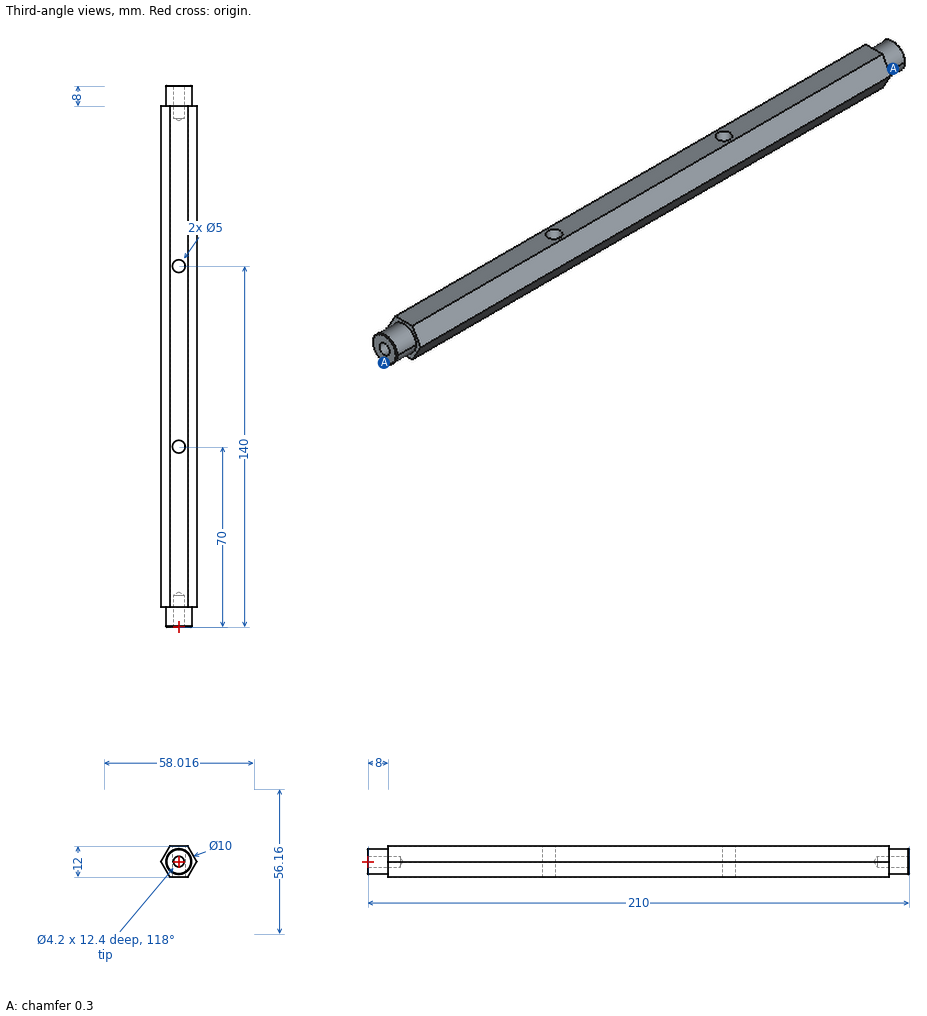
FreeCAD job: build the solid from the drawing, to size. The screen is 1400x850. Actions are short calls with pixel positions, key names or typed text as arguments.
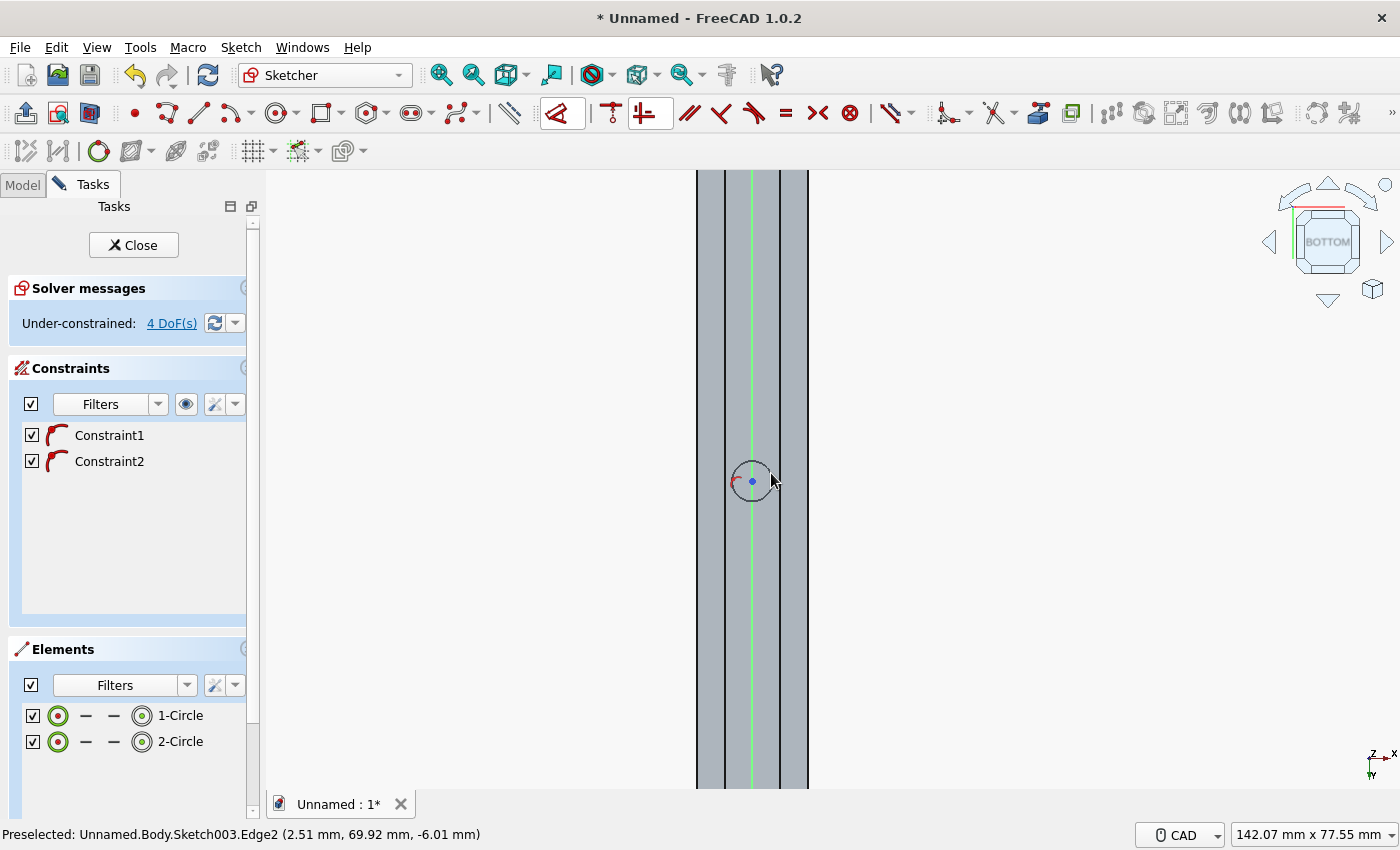
scroll(772, 474, down, 5)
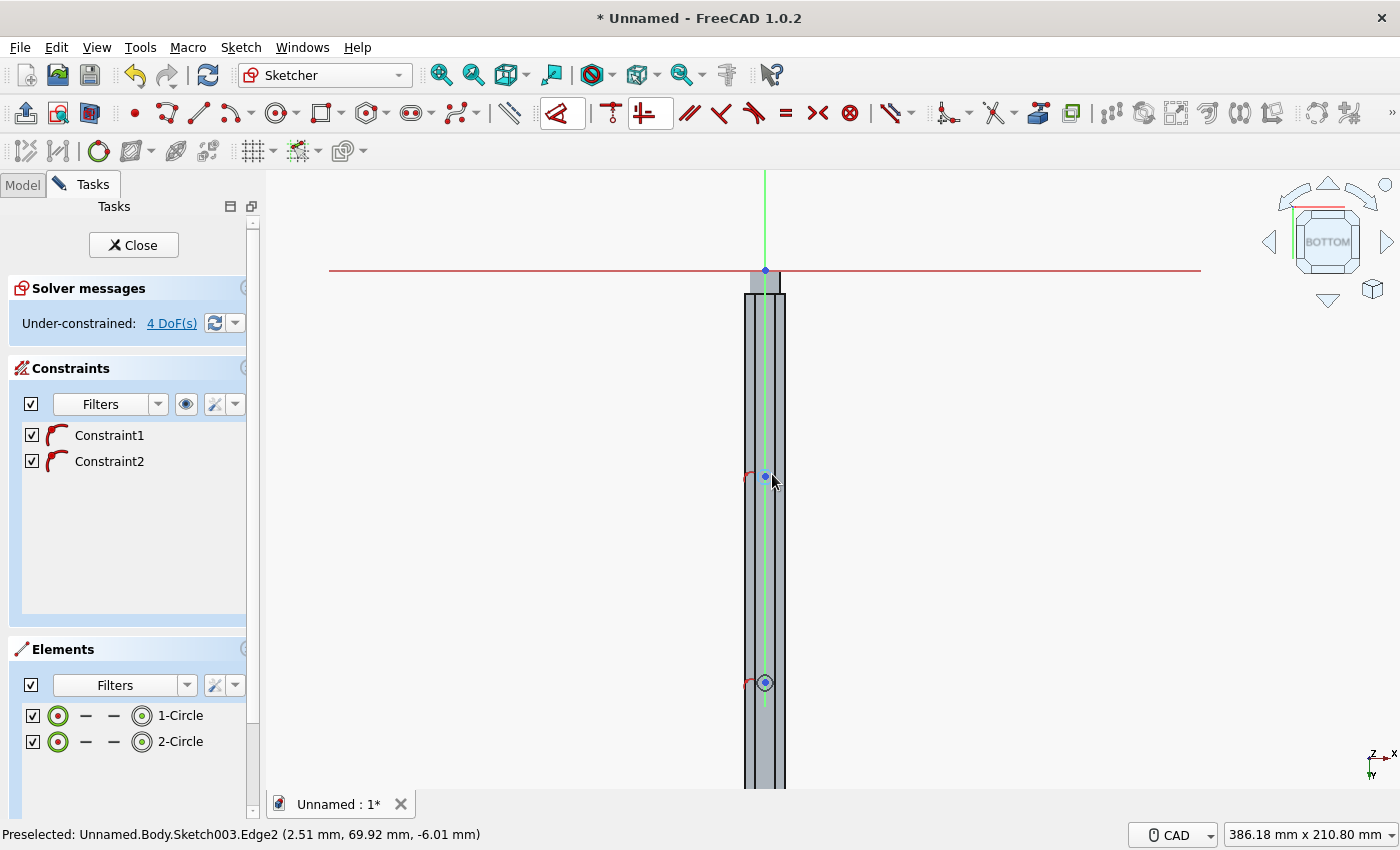
scroll(770, 678, up, 5)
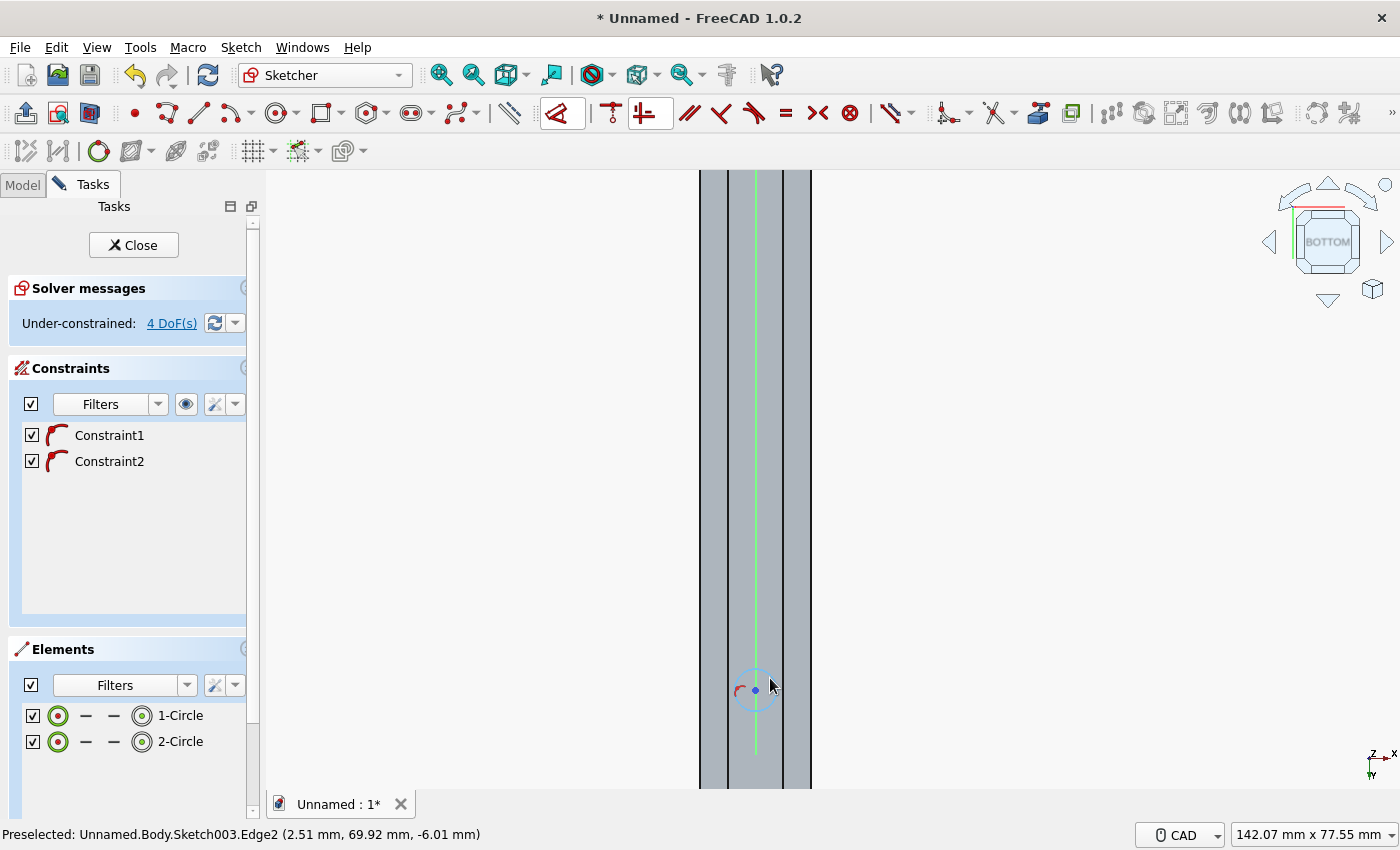
click(770, 675)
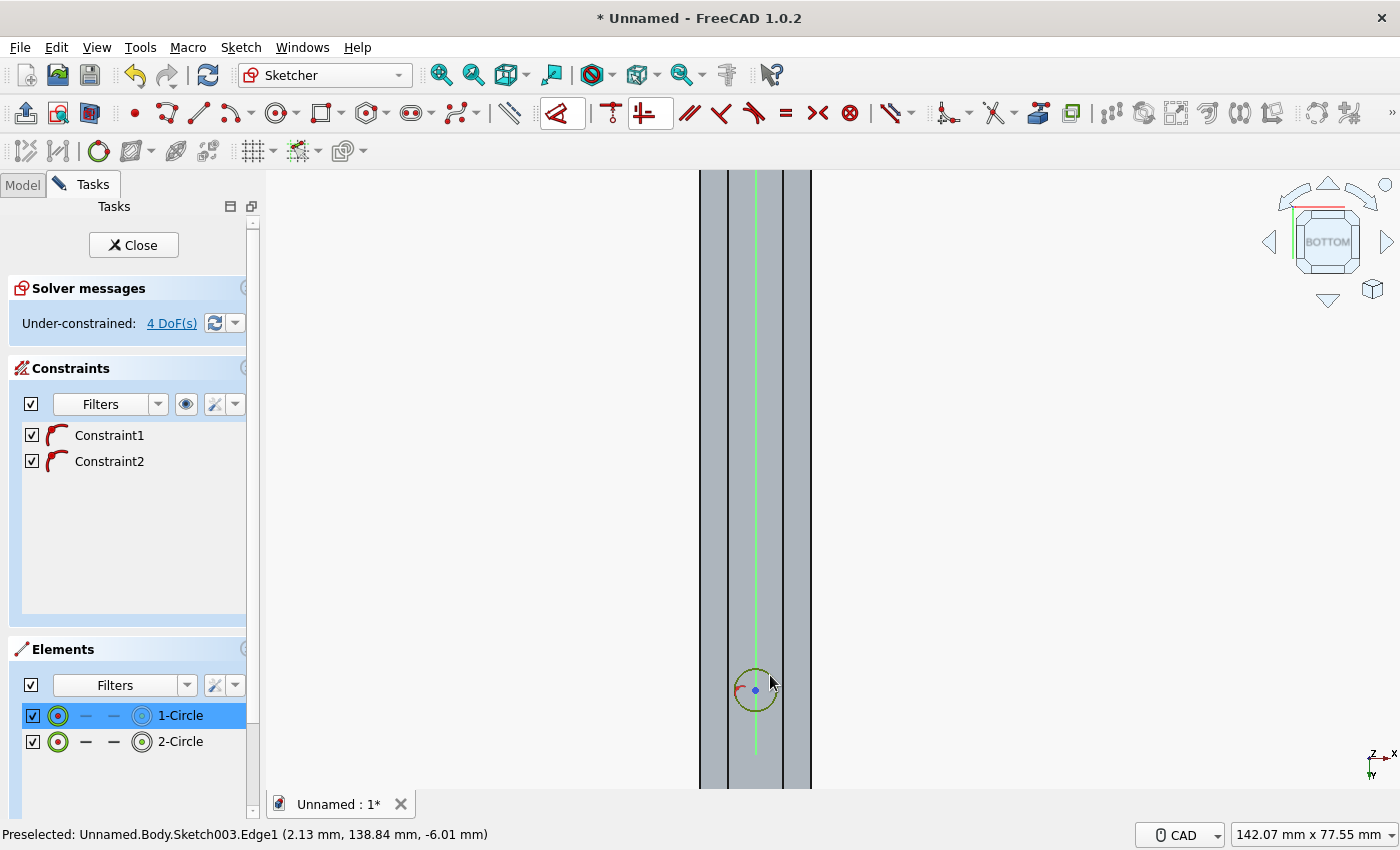
scroll(770, 678, down, 5)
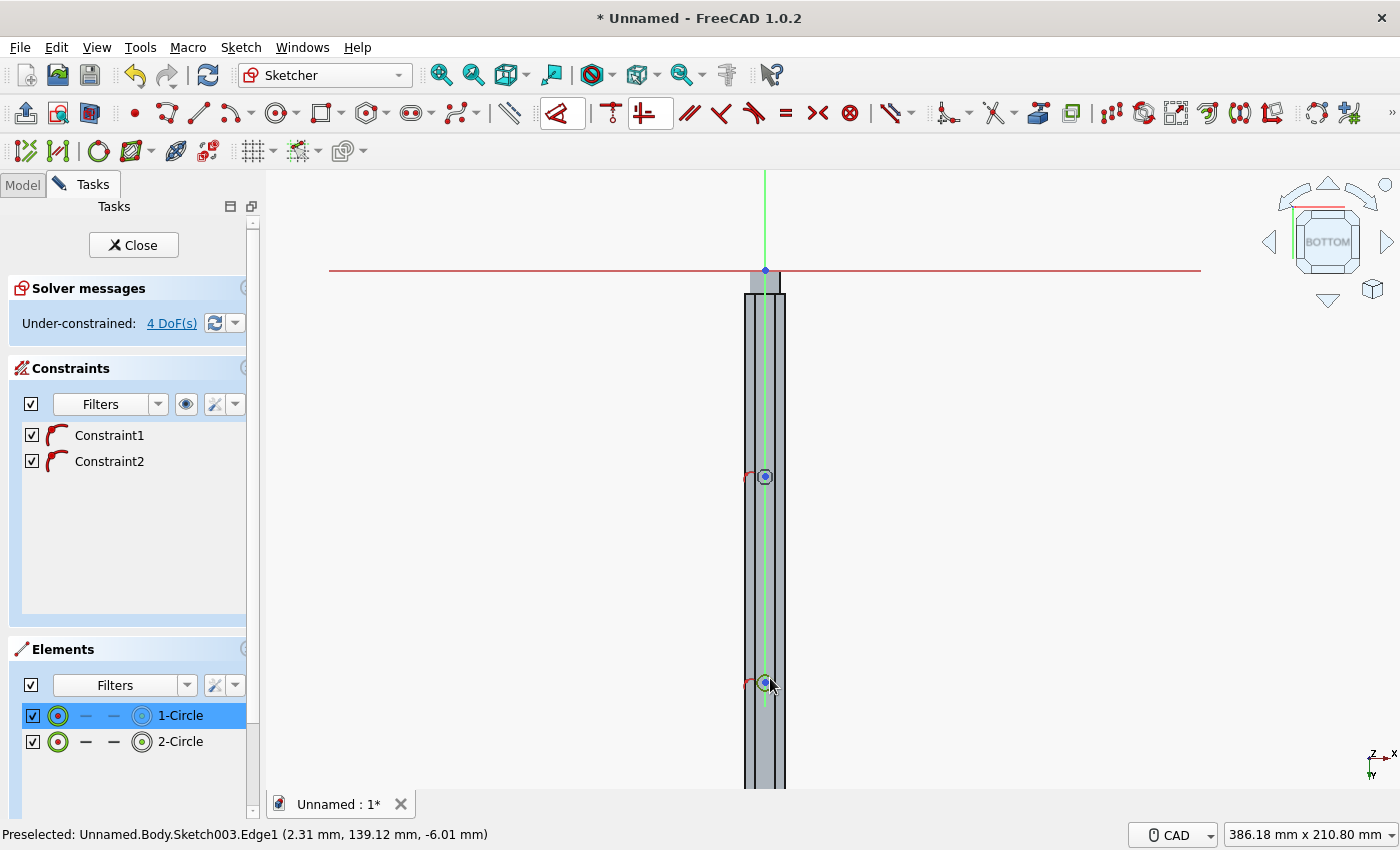
scroll(770, 472, up, 5)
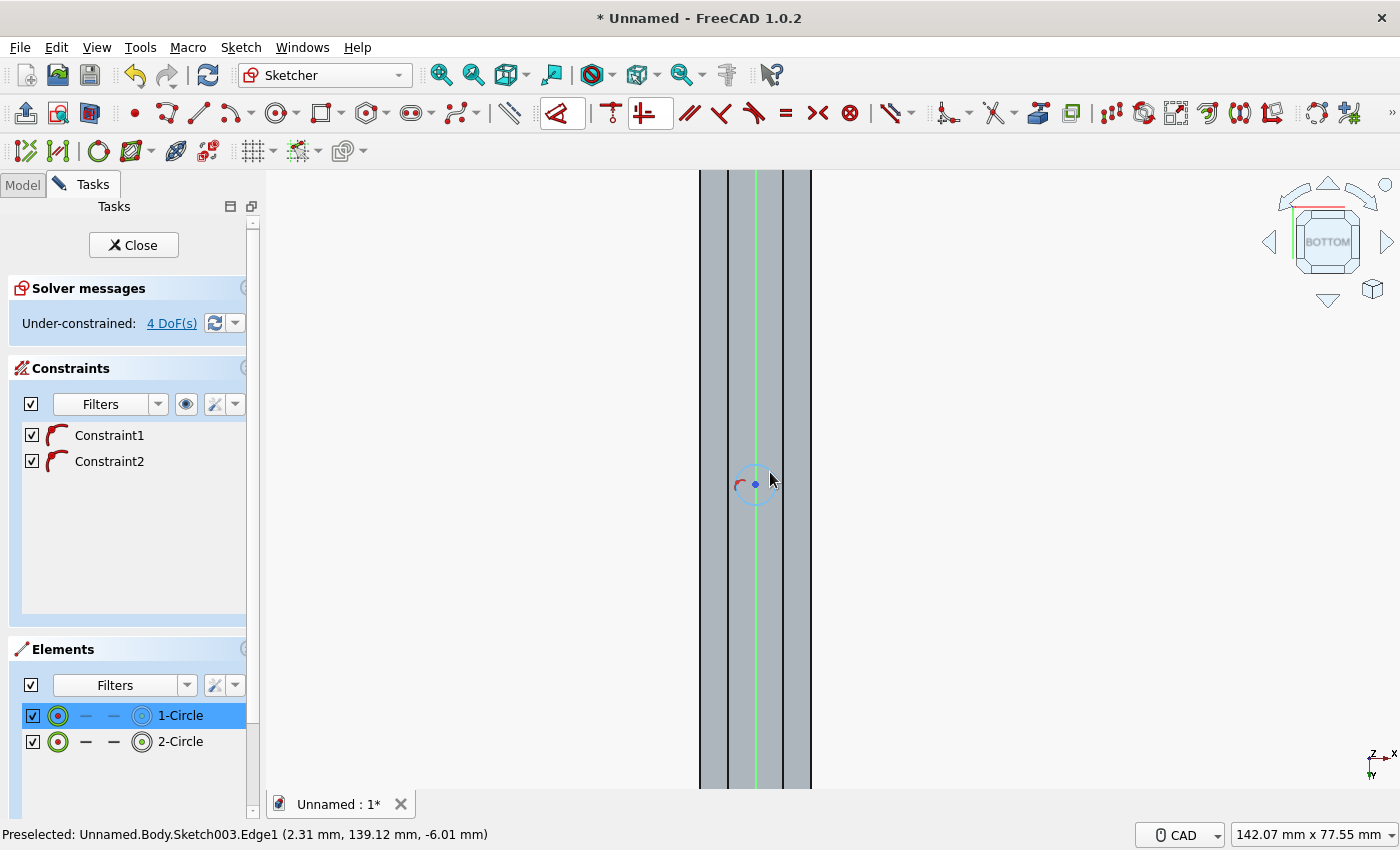
click(770, 470)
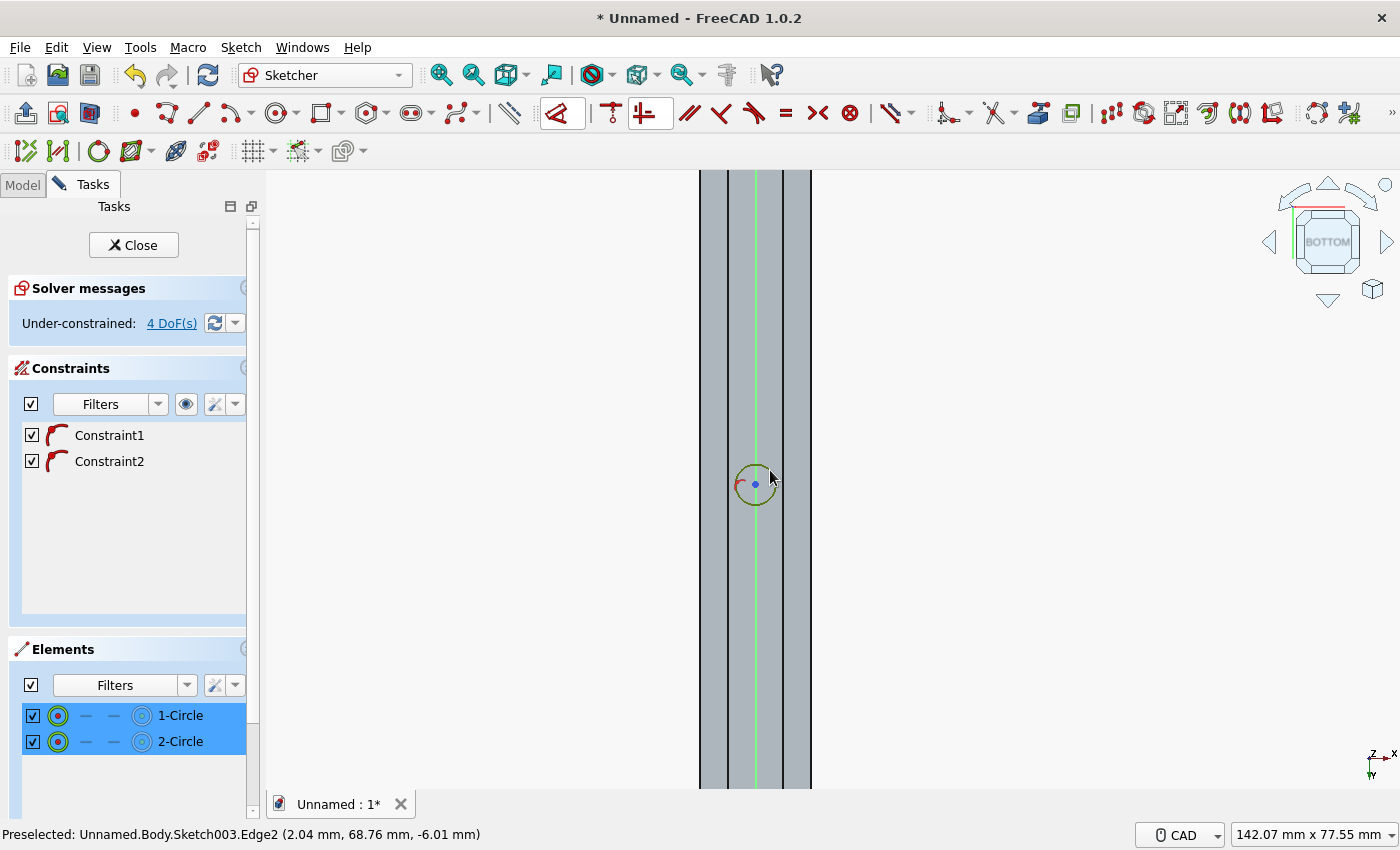
key(e)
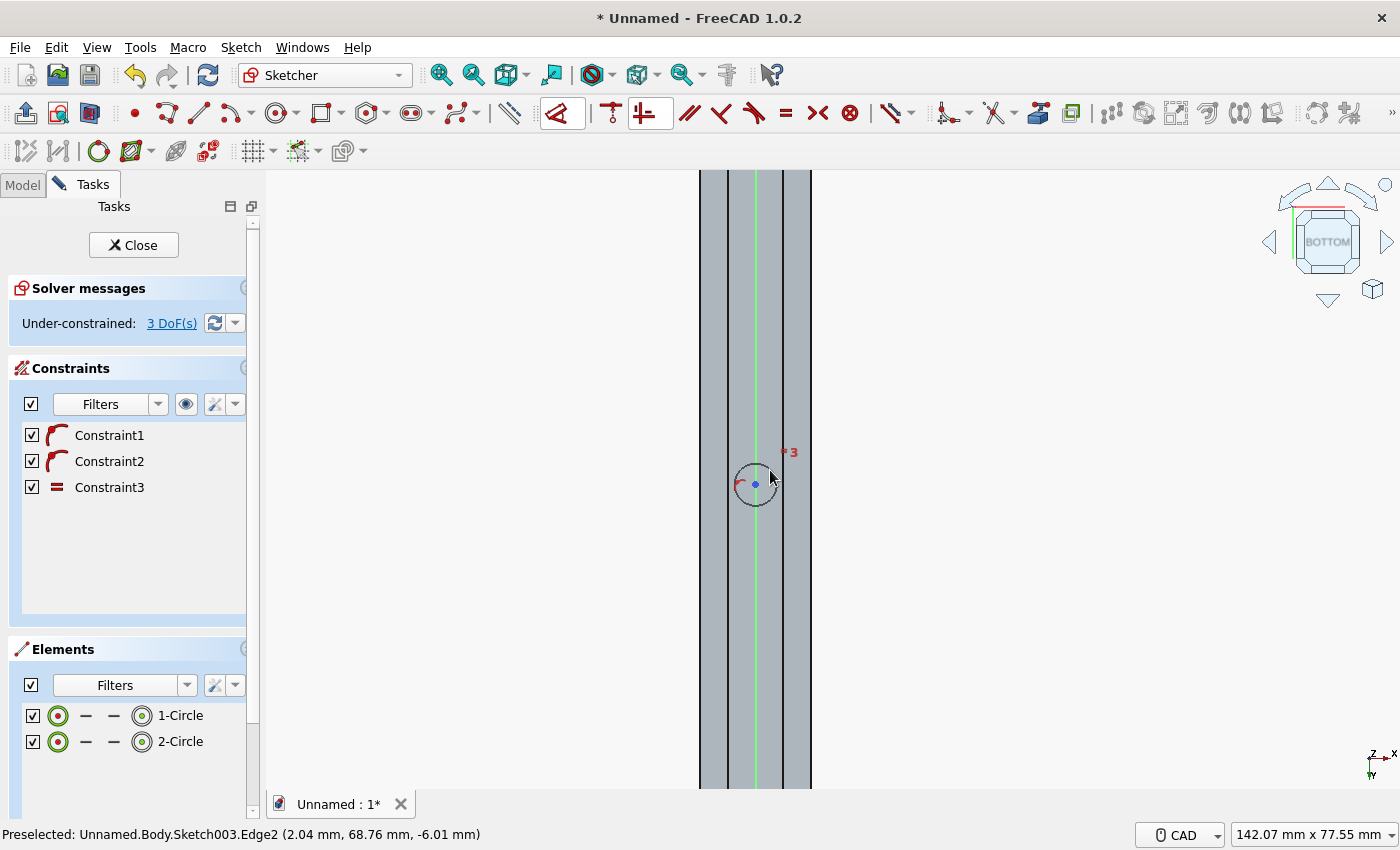
scroll(770, 472, down, 5)